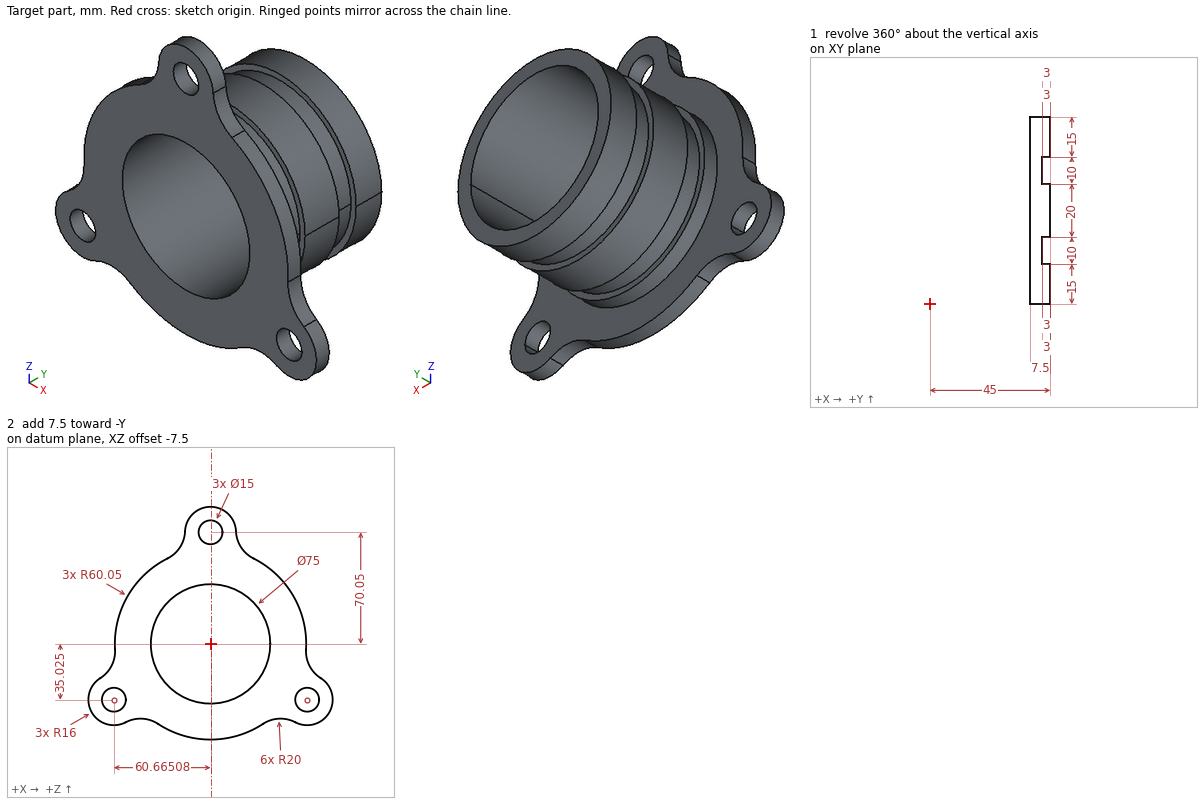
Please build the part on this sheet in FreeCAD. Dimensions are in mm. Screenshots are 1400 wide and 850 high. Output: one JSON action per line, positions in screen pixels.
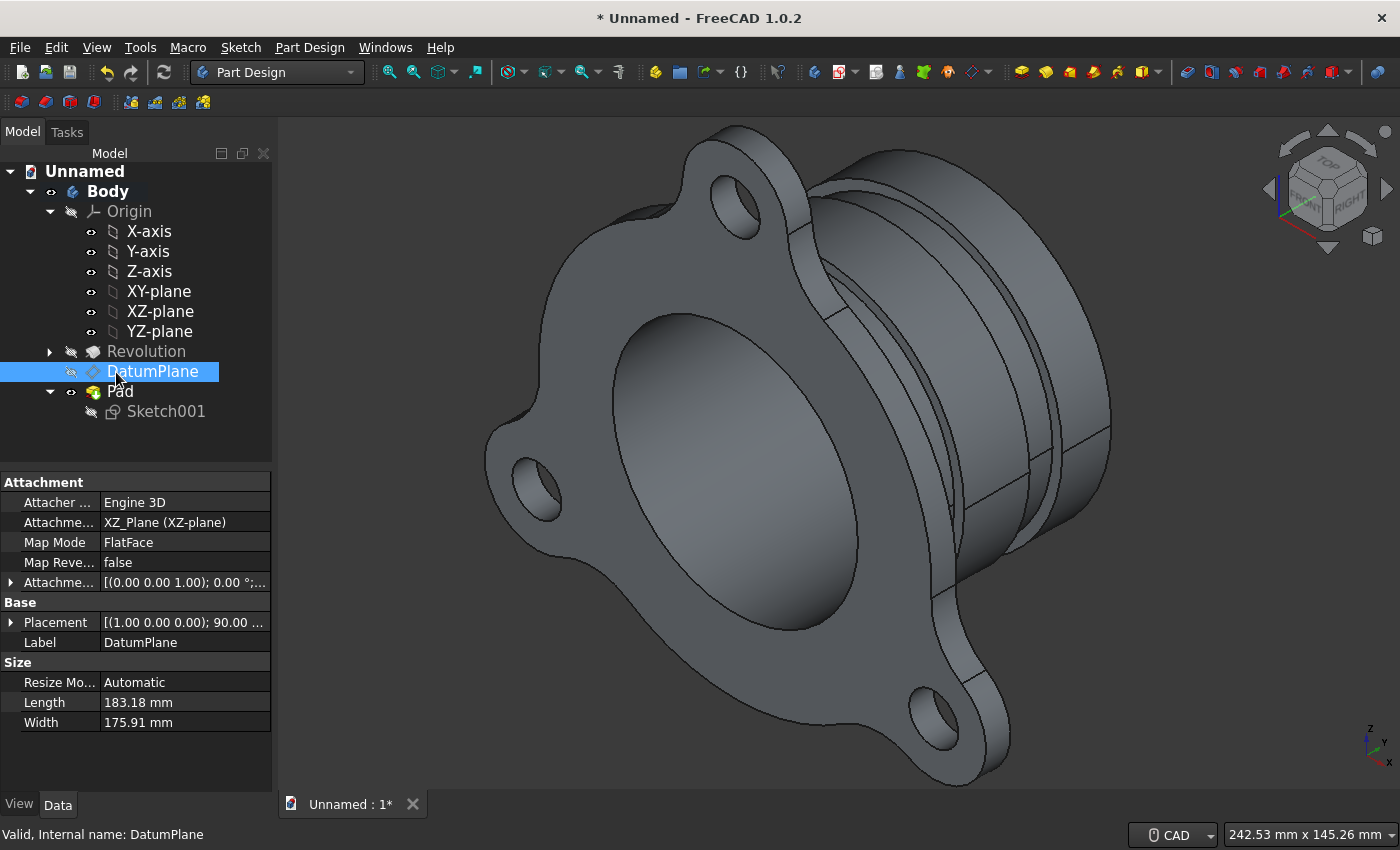
{"action": "left_click", "coordinate": [390, 72]}